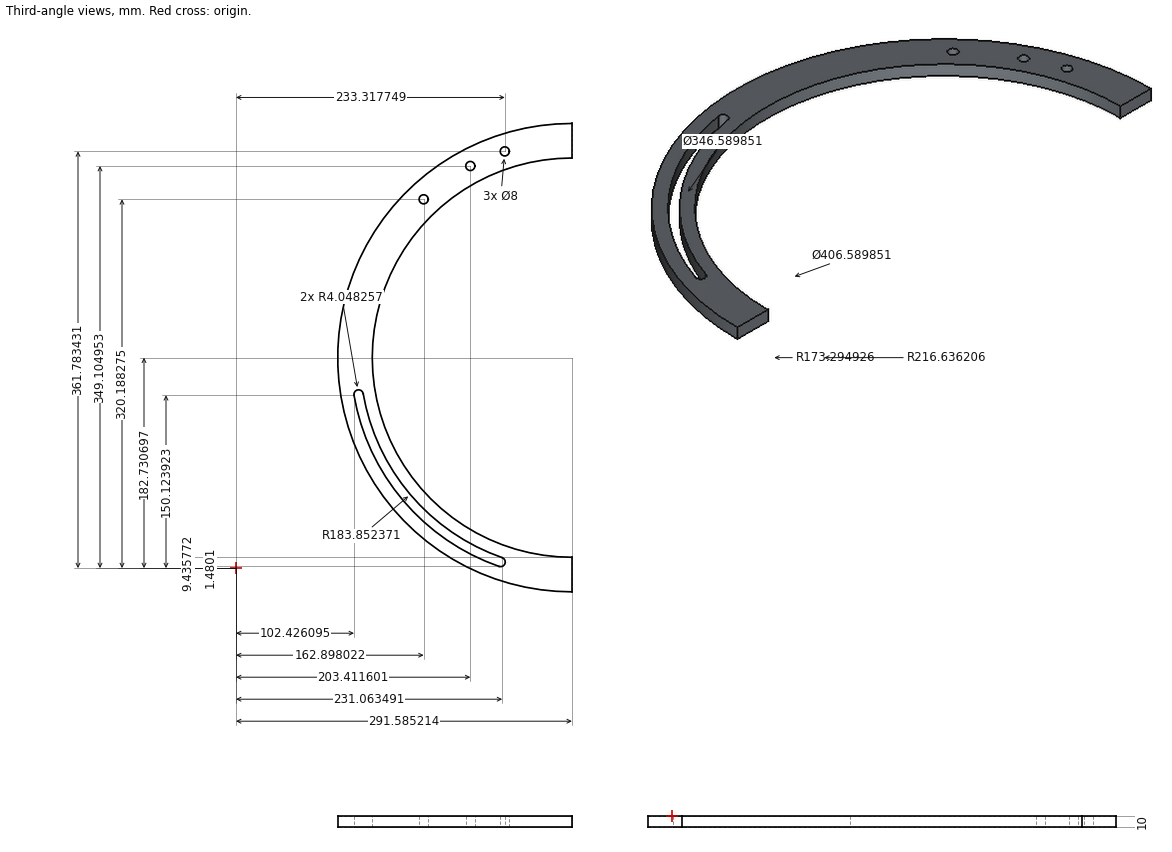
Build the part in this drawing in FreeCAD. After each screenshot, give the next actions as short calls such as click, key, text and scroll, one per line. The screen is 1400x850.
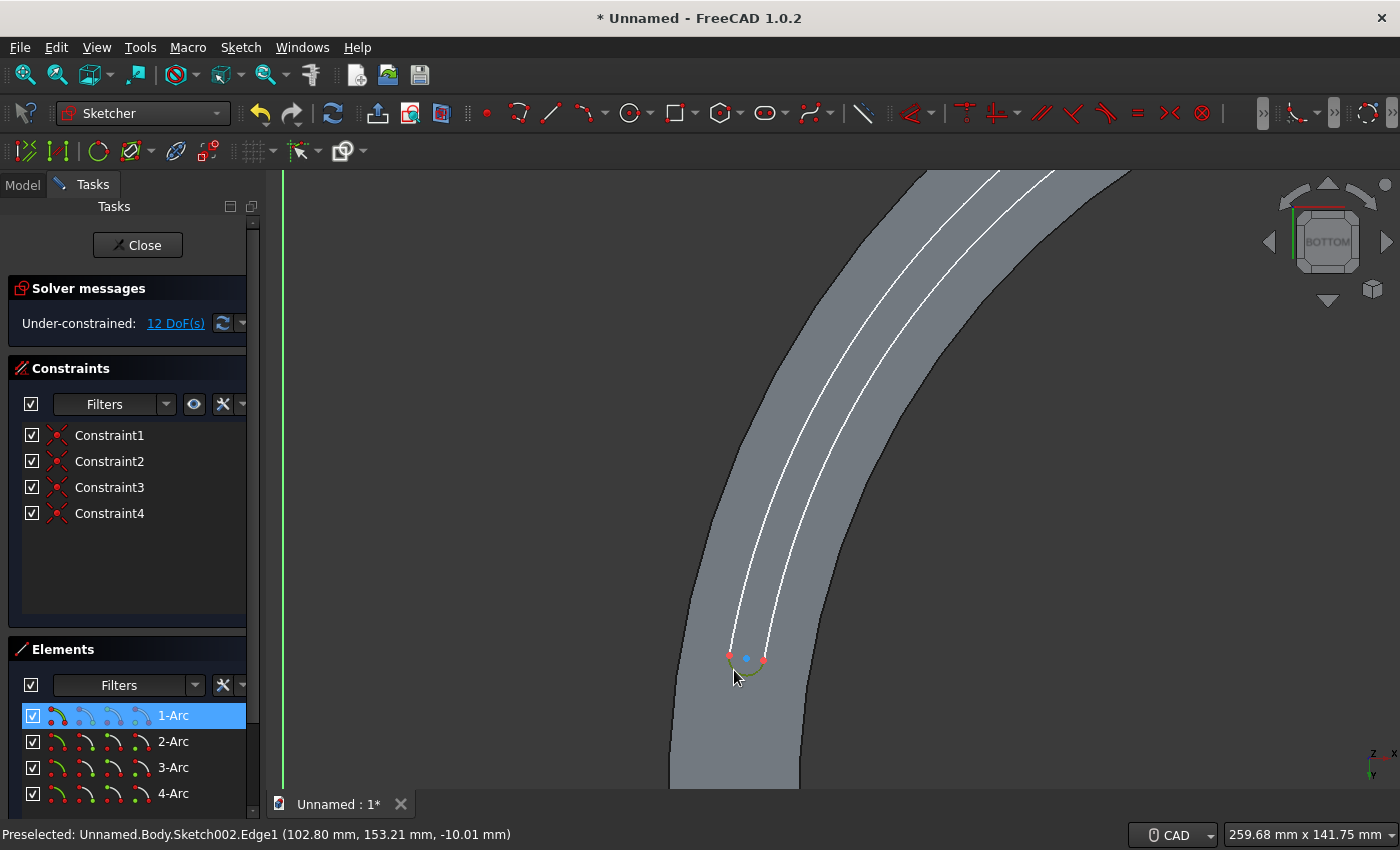
click(847, 419)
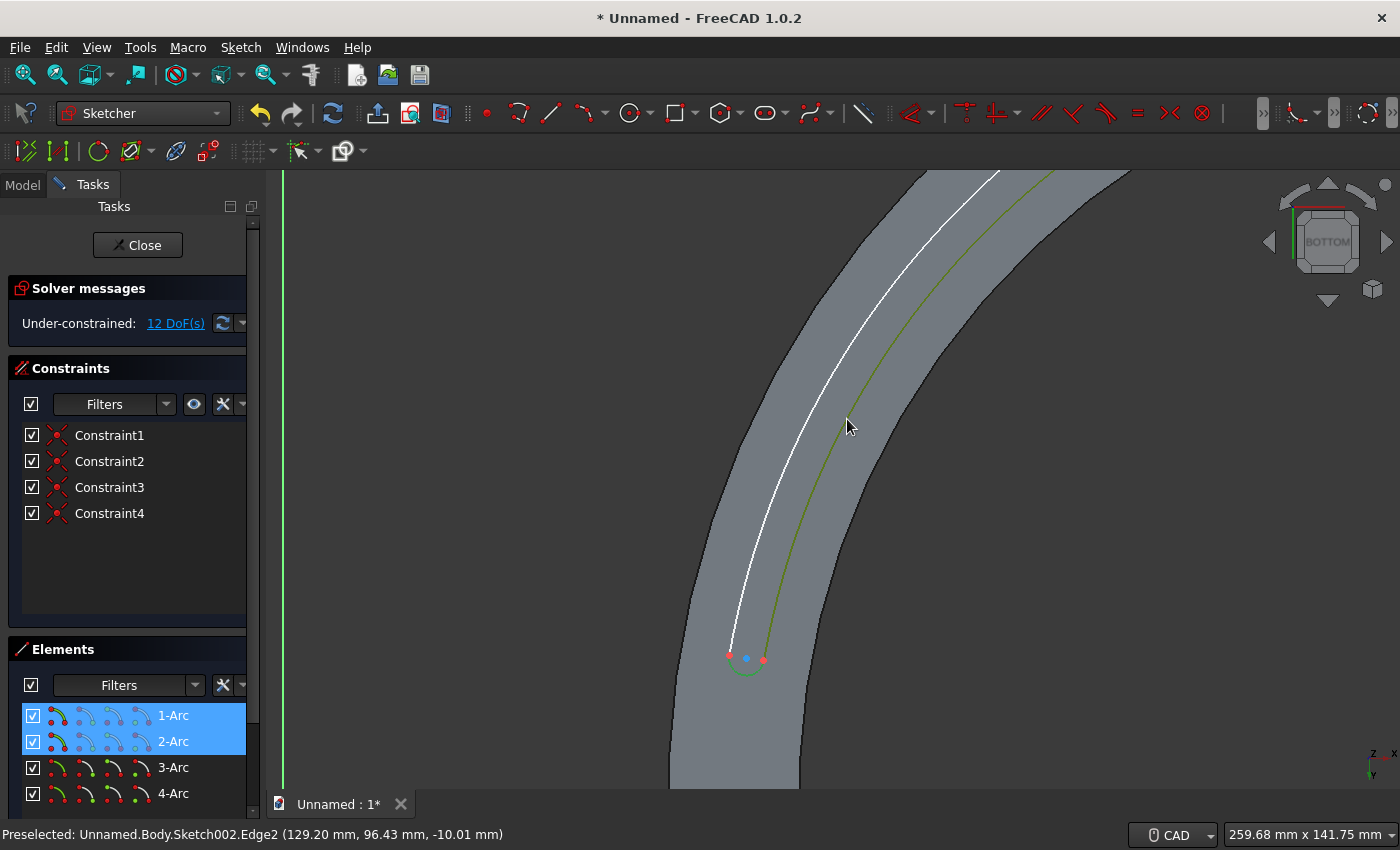
click(1106, 114)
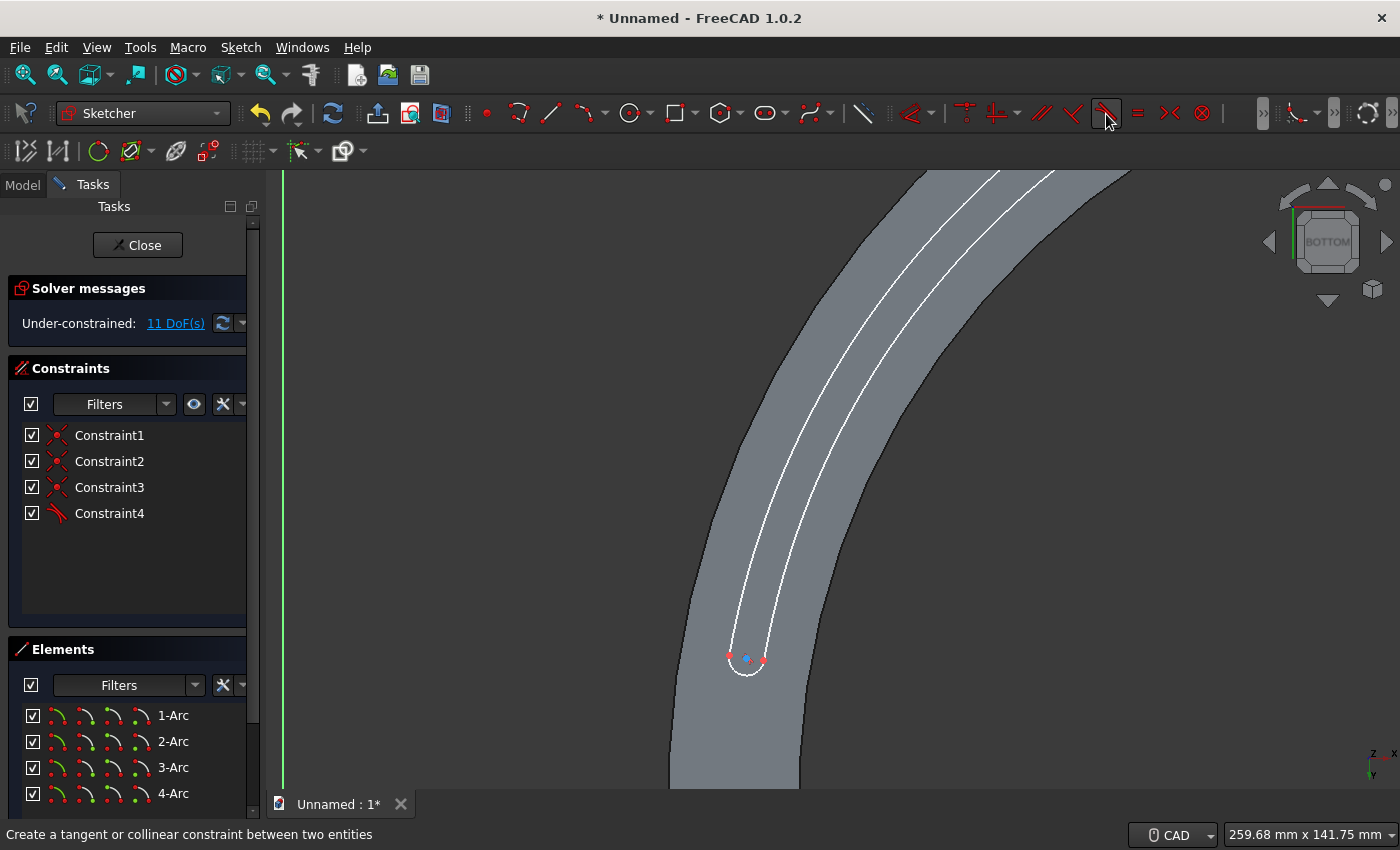
click(734, 670)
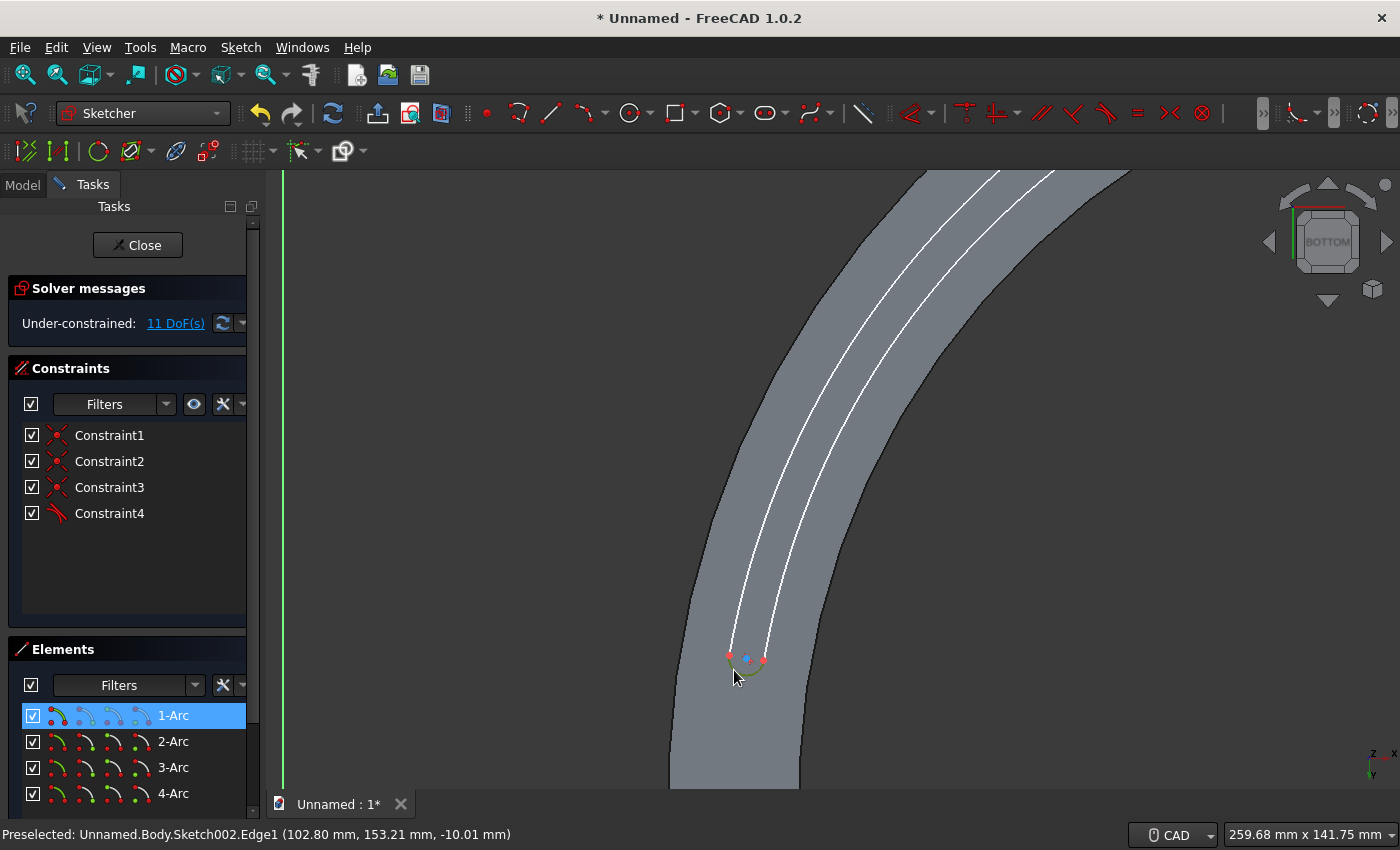
click(816, 403)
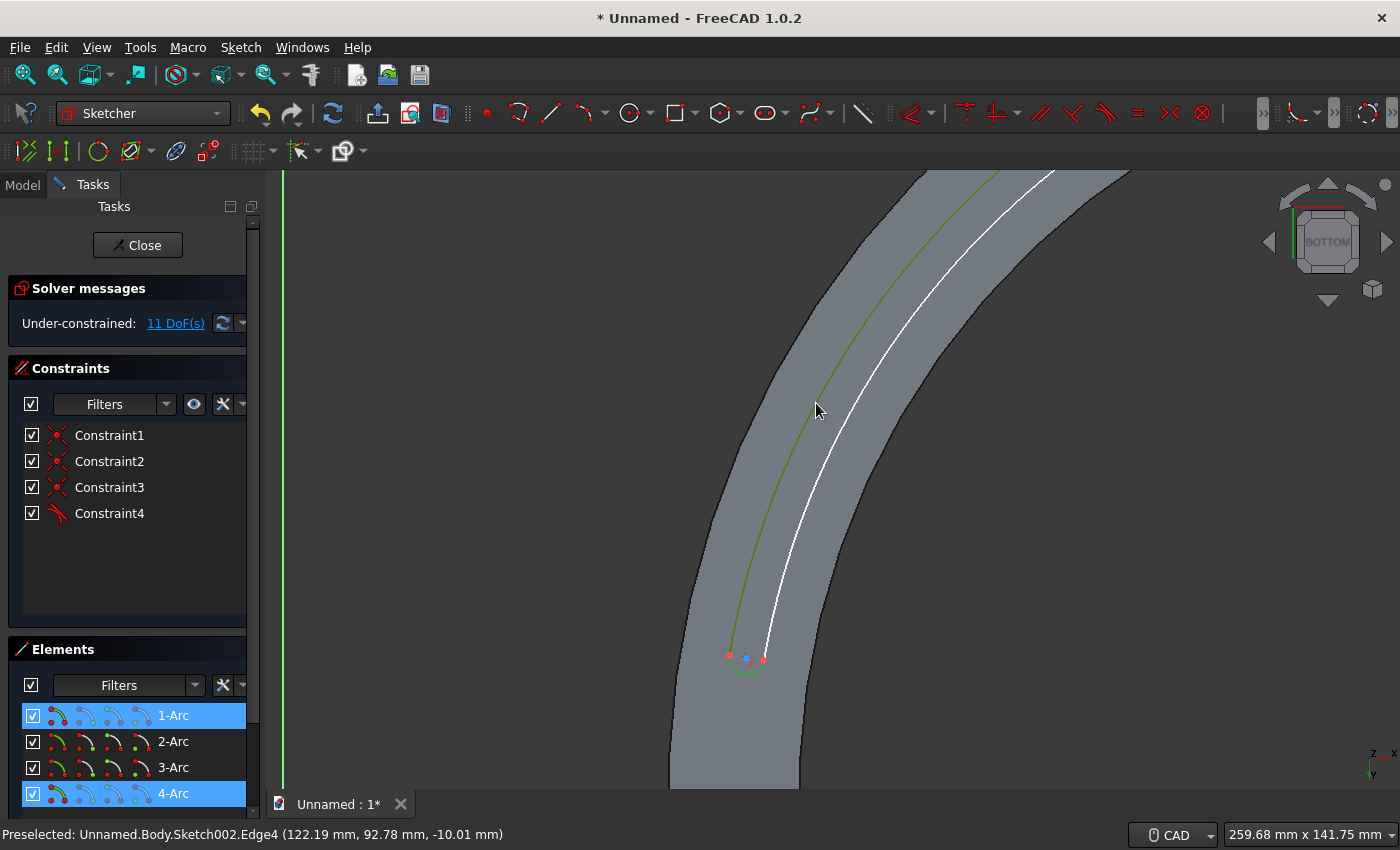
key(t)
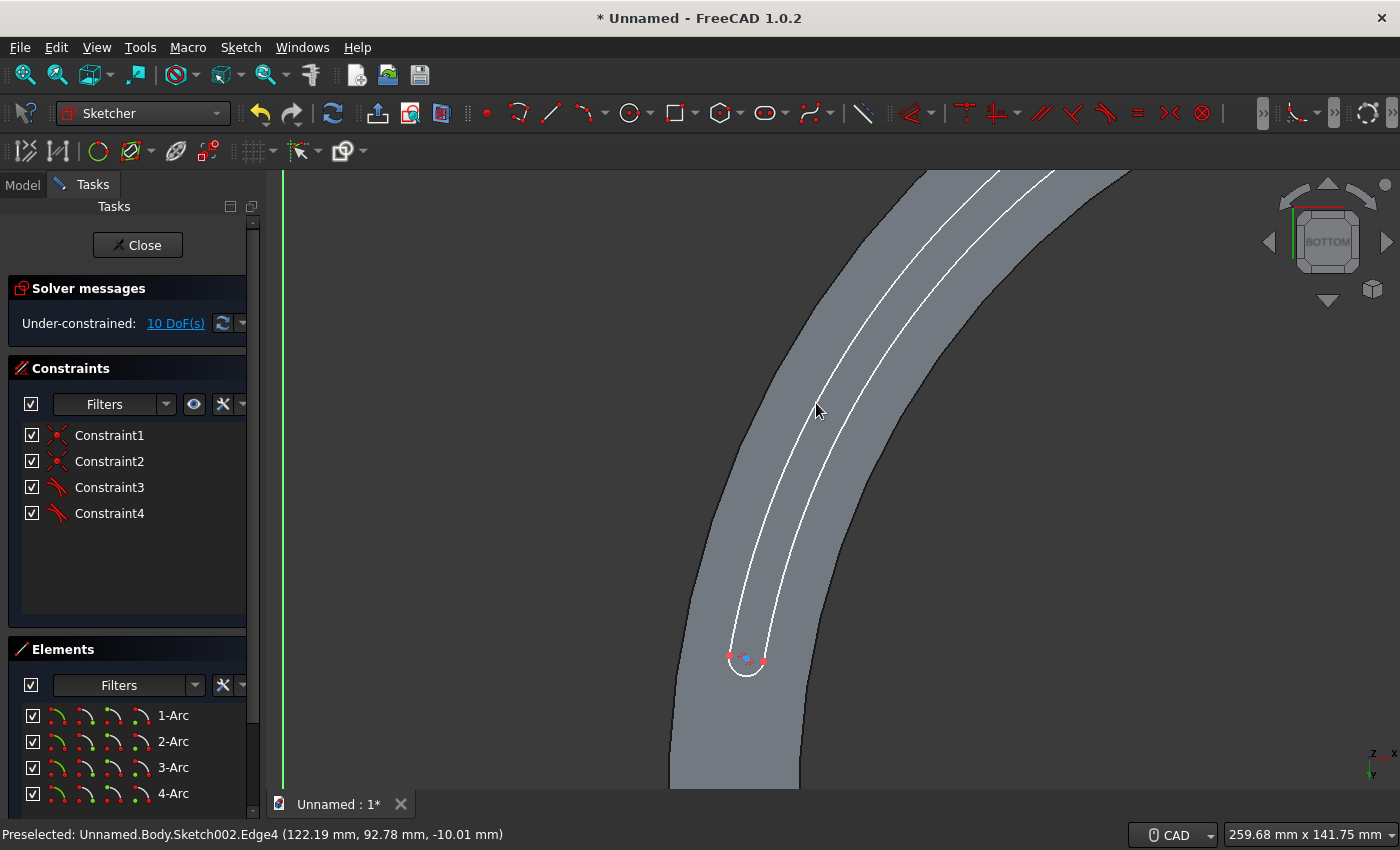
click(847, 419)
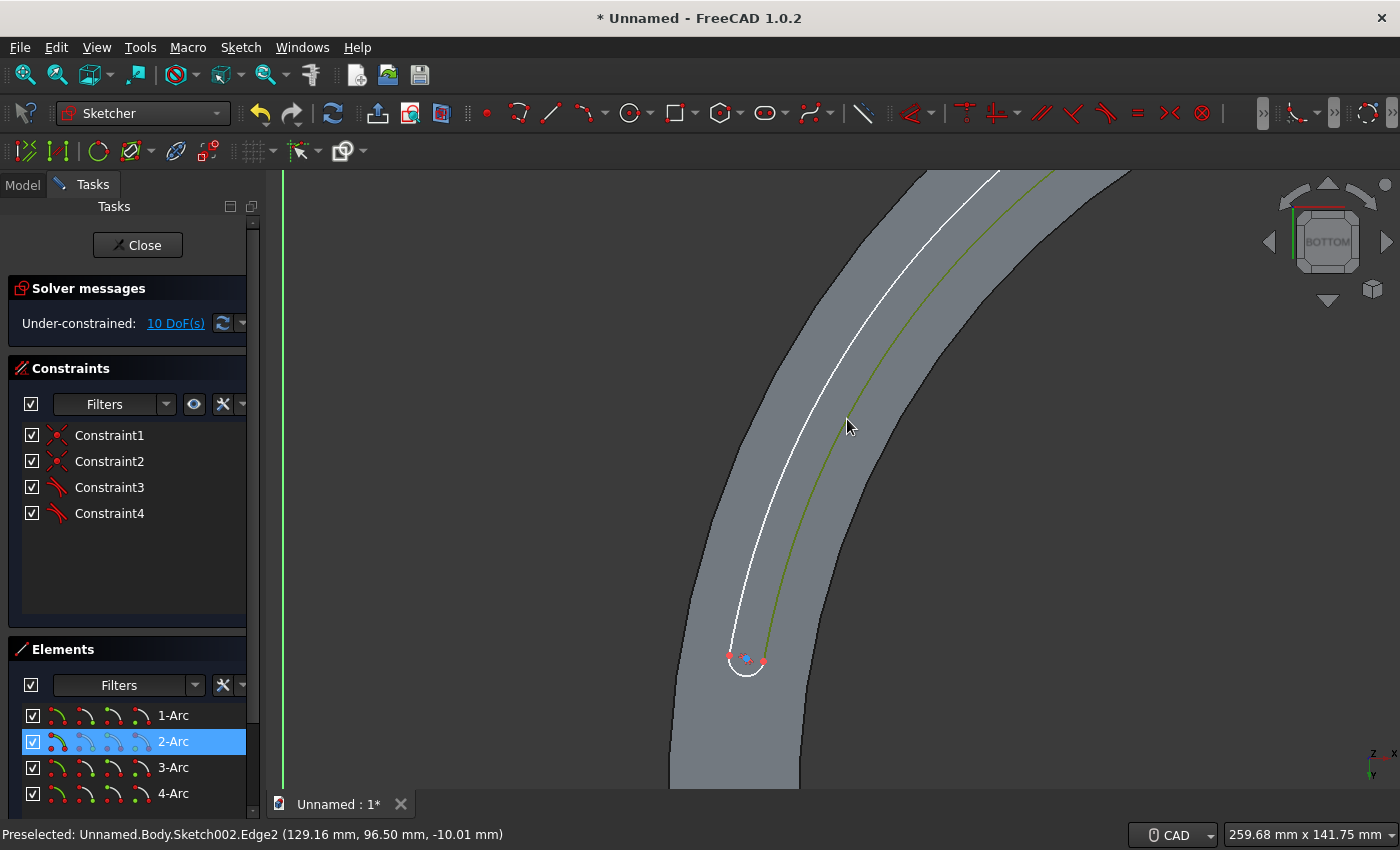
scroll(730, 654, down, 3)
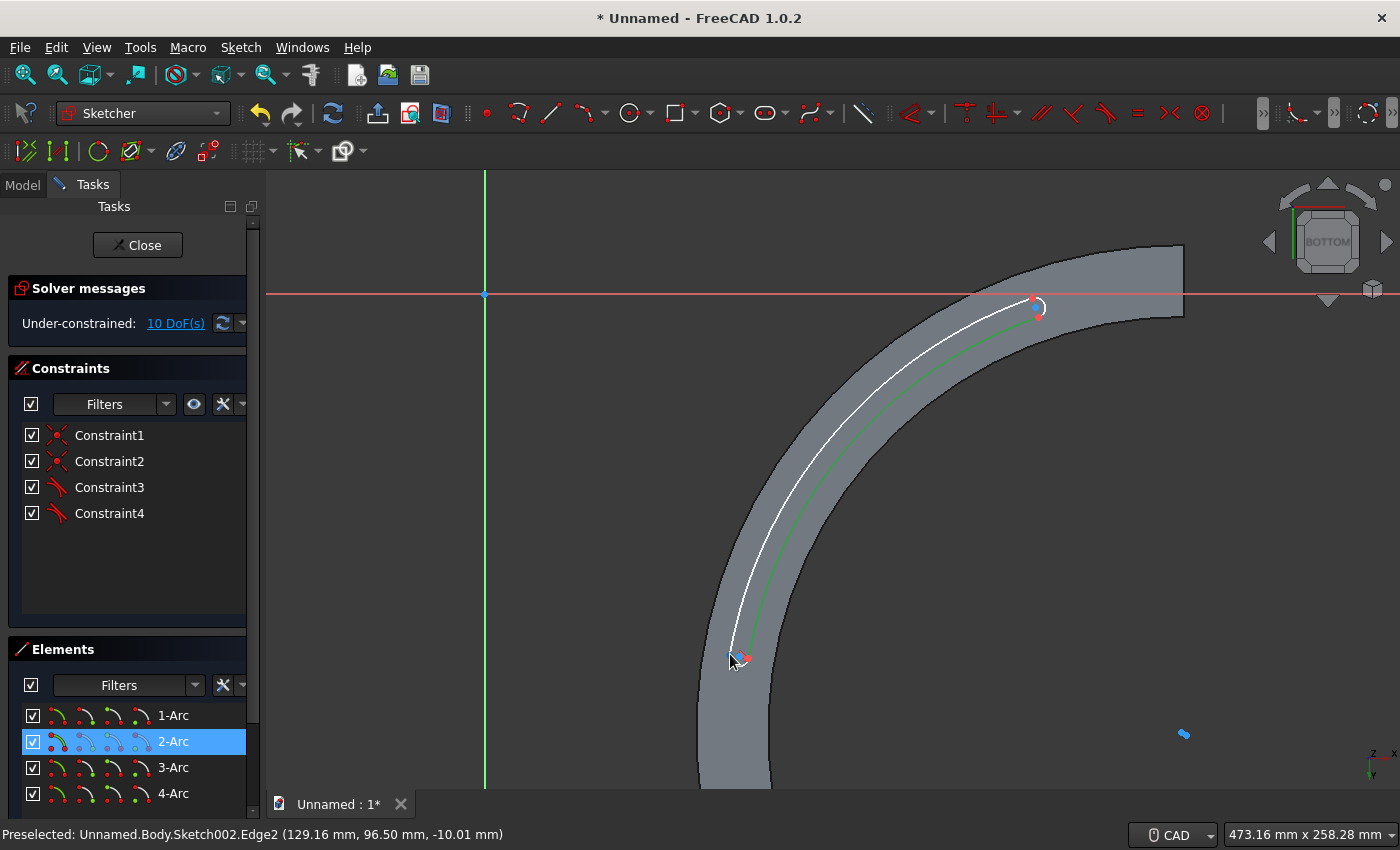
scroll(1045, 310, up, 3)